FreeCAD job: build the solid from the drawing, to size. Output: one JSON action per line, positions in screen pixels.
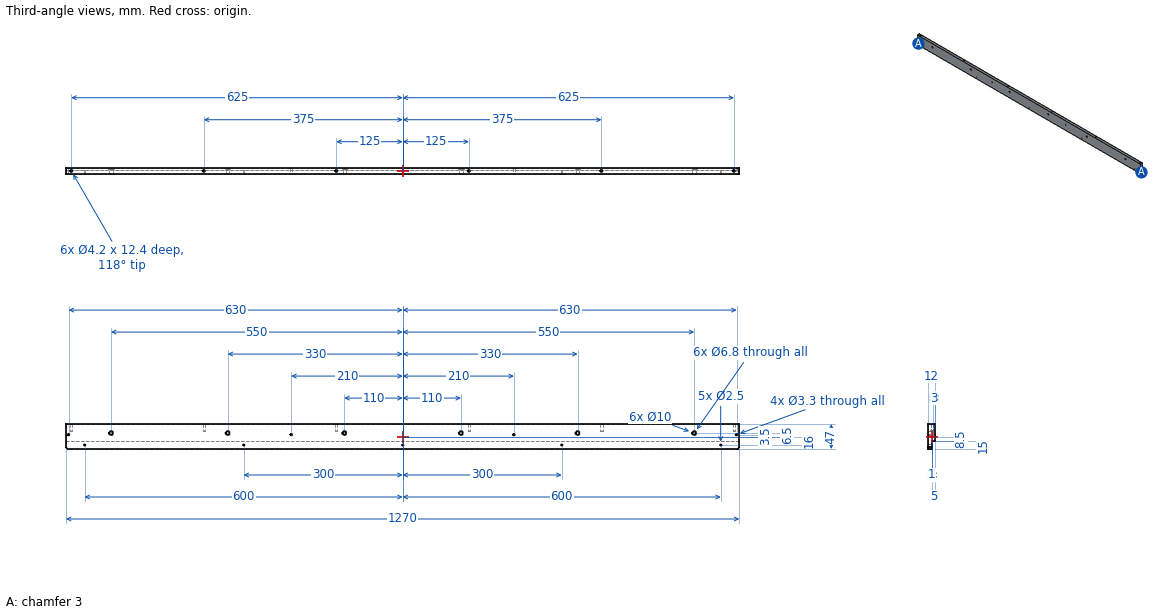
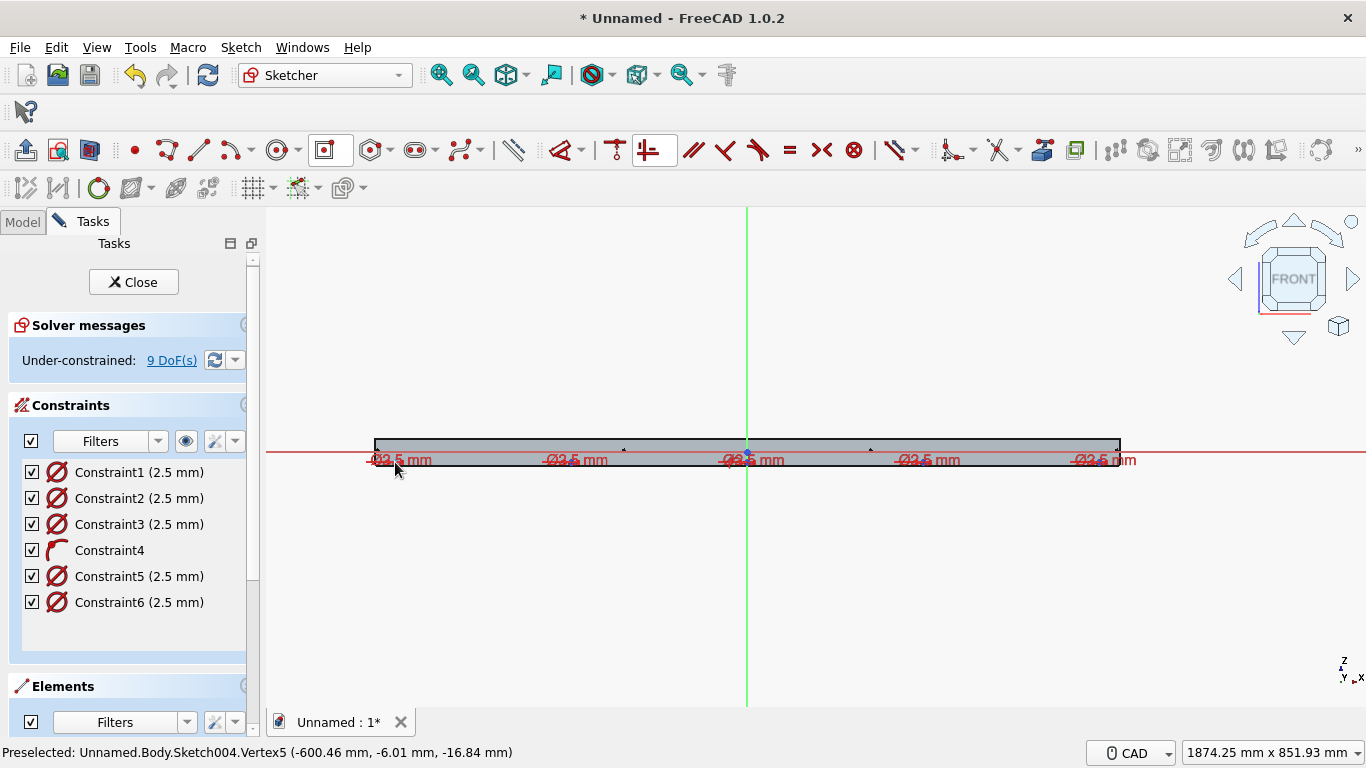
{"action": "left_click", "coordinate": [1100, 462]}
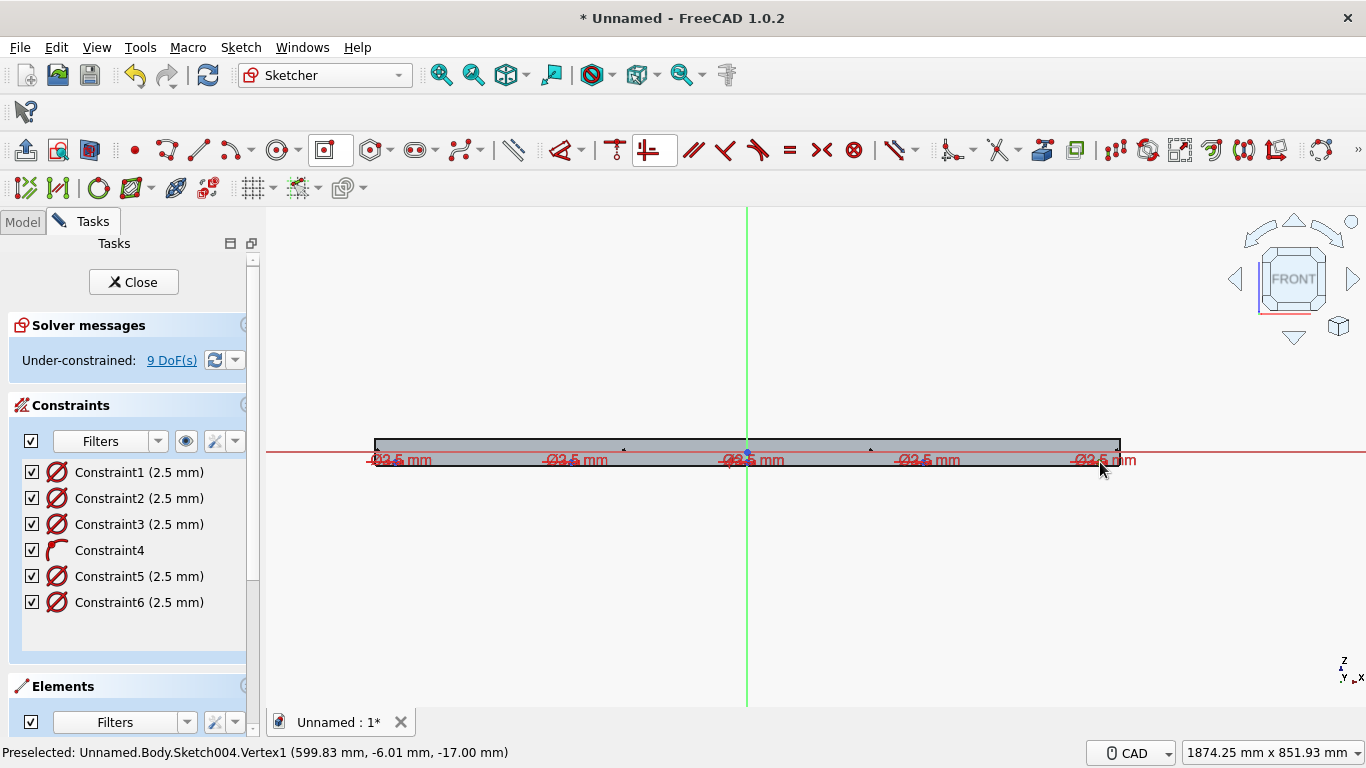
{"action": "left_click", "coordinate": [923, 462]}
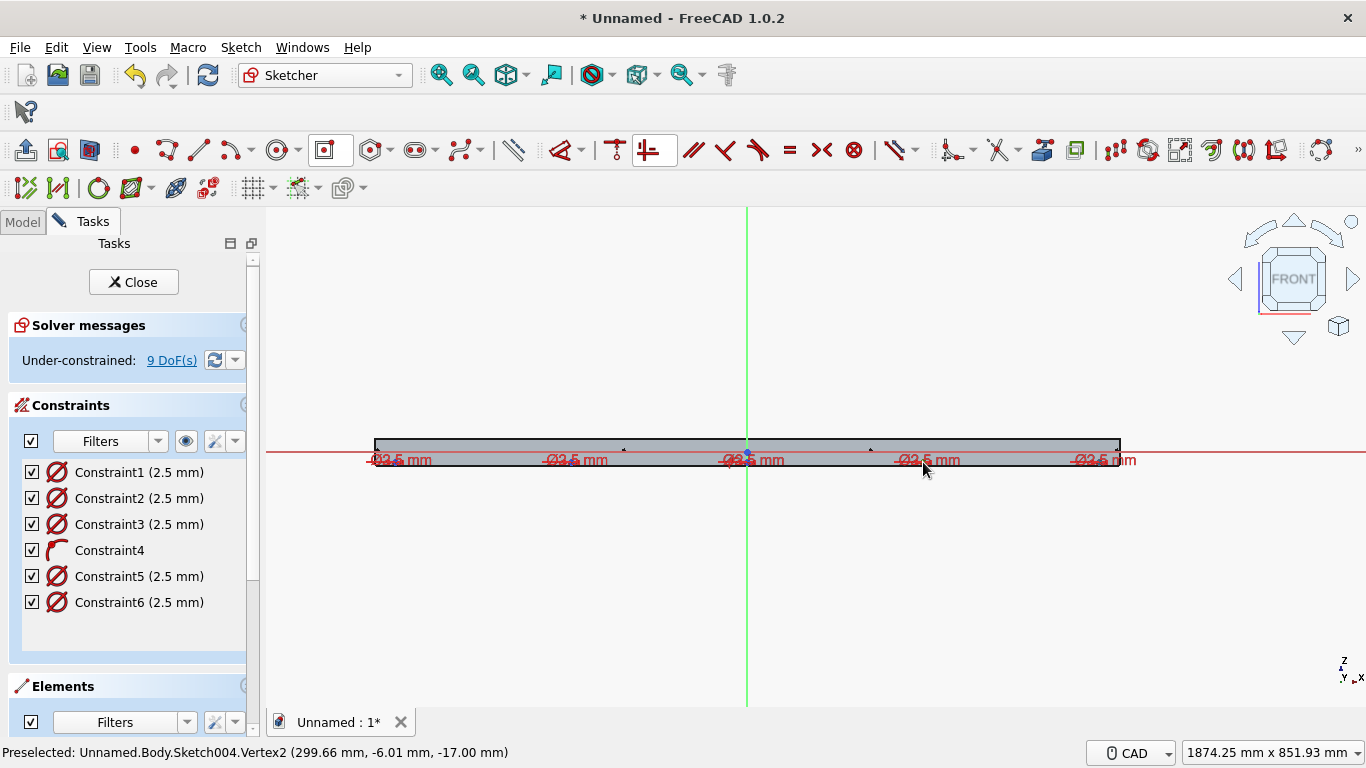
{"action": "key", "text": "h"}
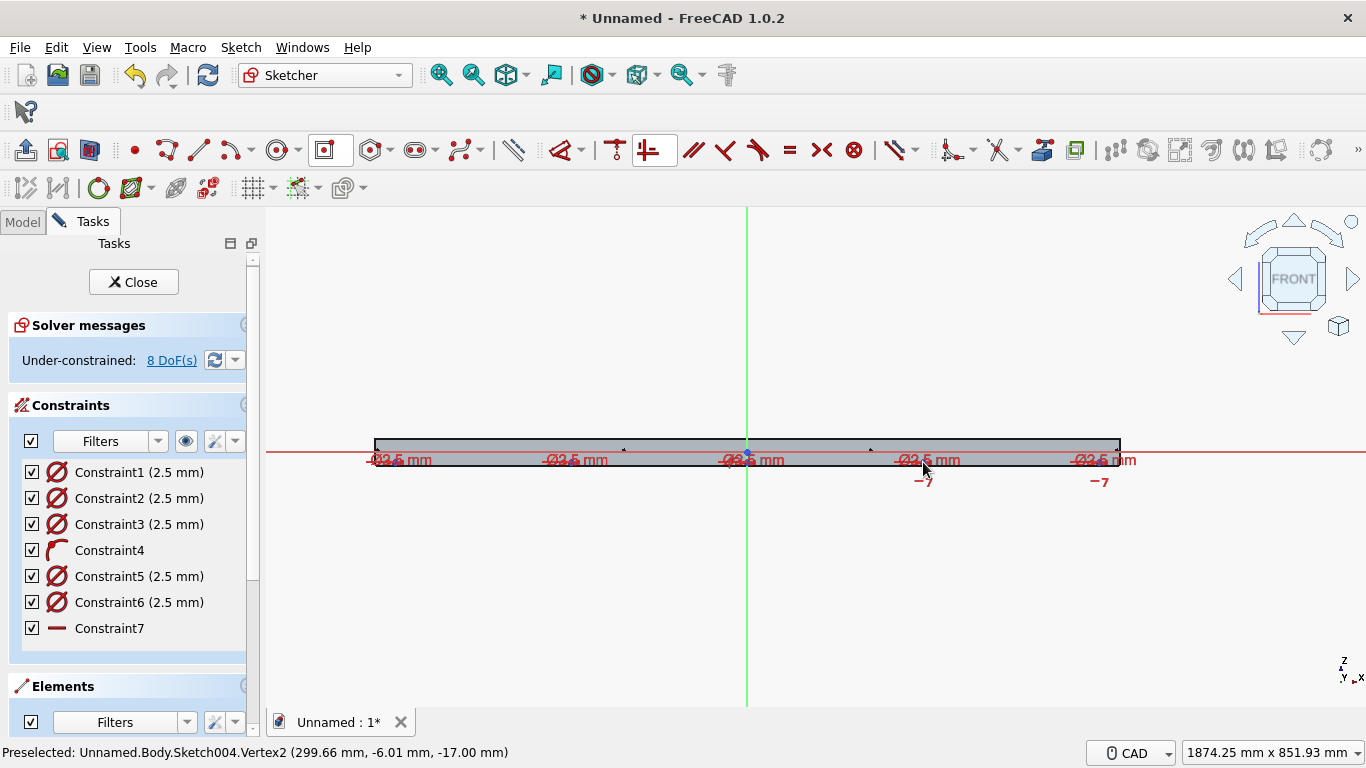
{"action": "left_click", "coordinate": [923, 462]}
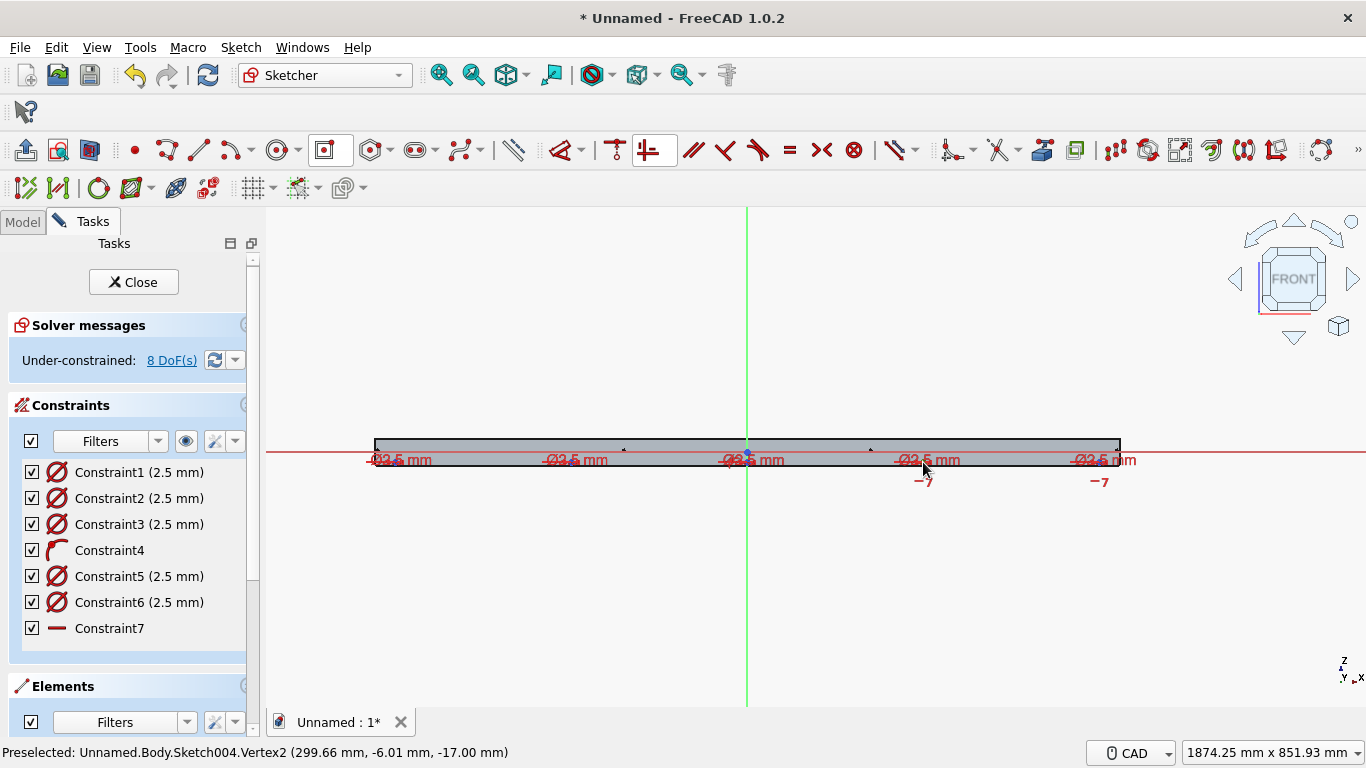
{"action": "scroll", "coordinate": [747, 462], "scroll_direction": "up", "scroll_amount": 2}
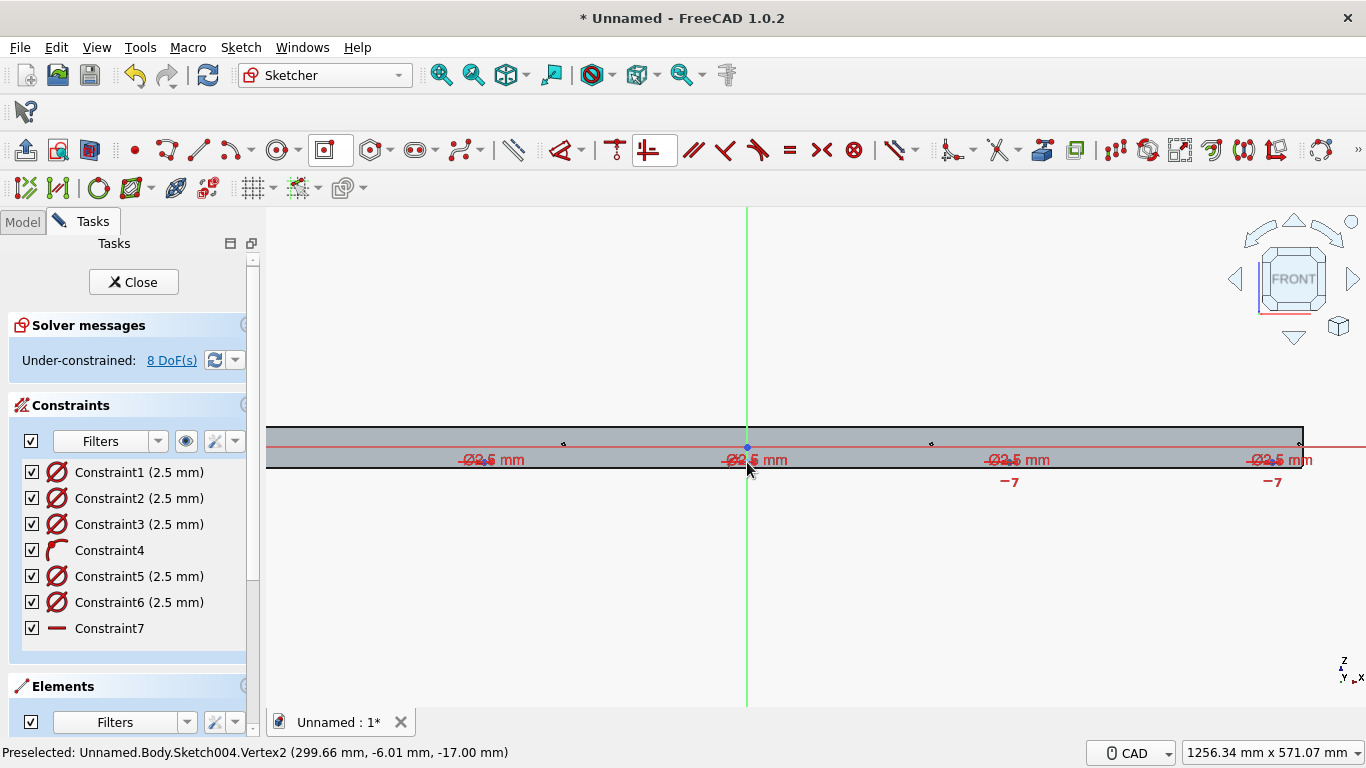
{"action": "left_click", "coordinate": [747, 462]}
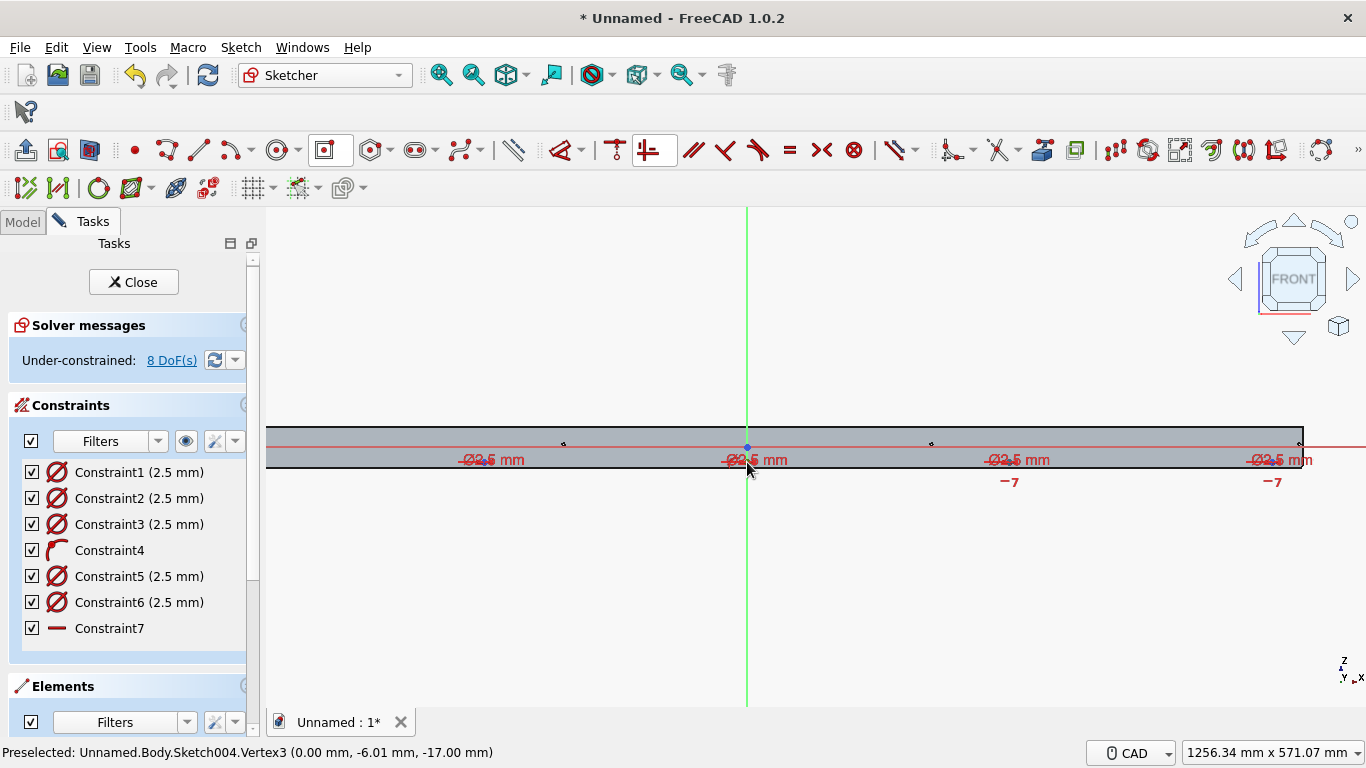
{"action": "left_click", "coordinate": [672, 150]}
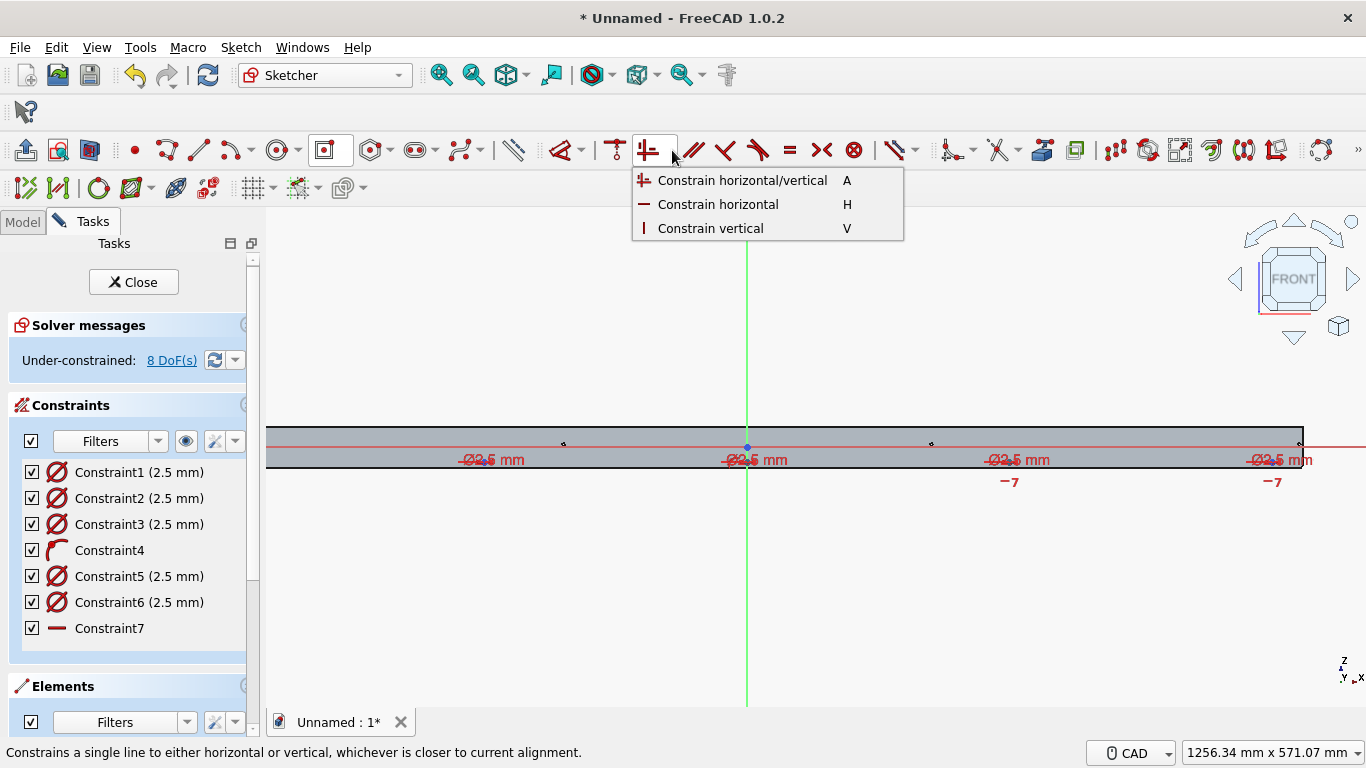
{"action": "left_click", "coordinate": [768, 204]}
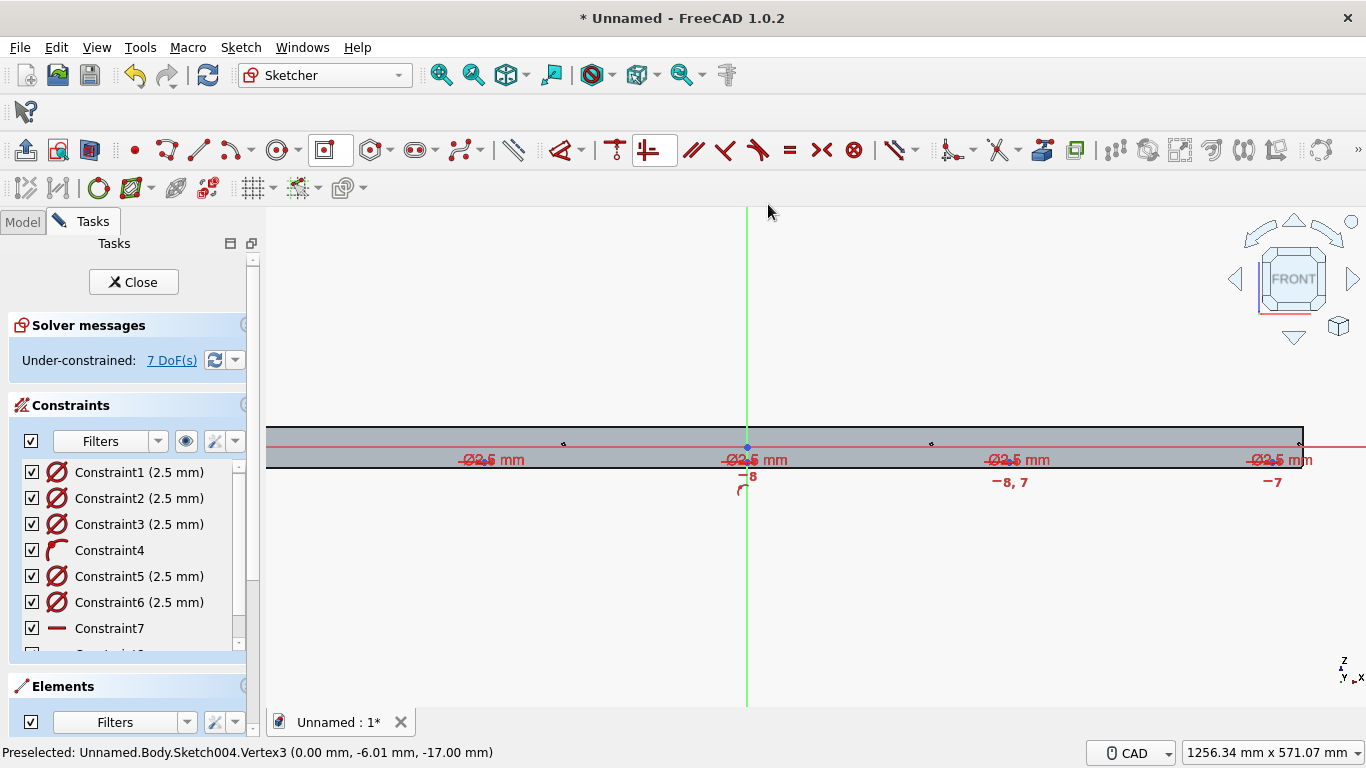
{"action": "left_click", "coordinate": [747, 462]}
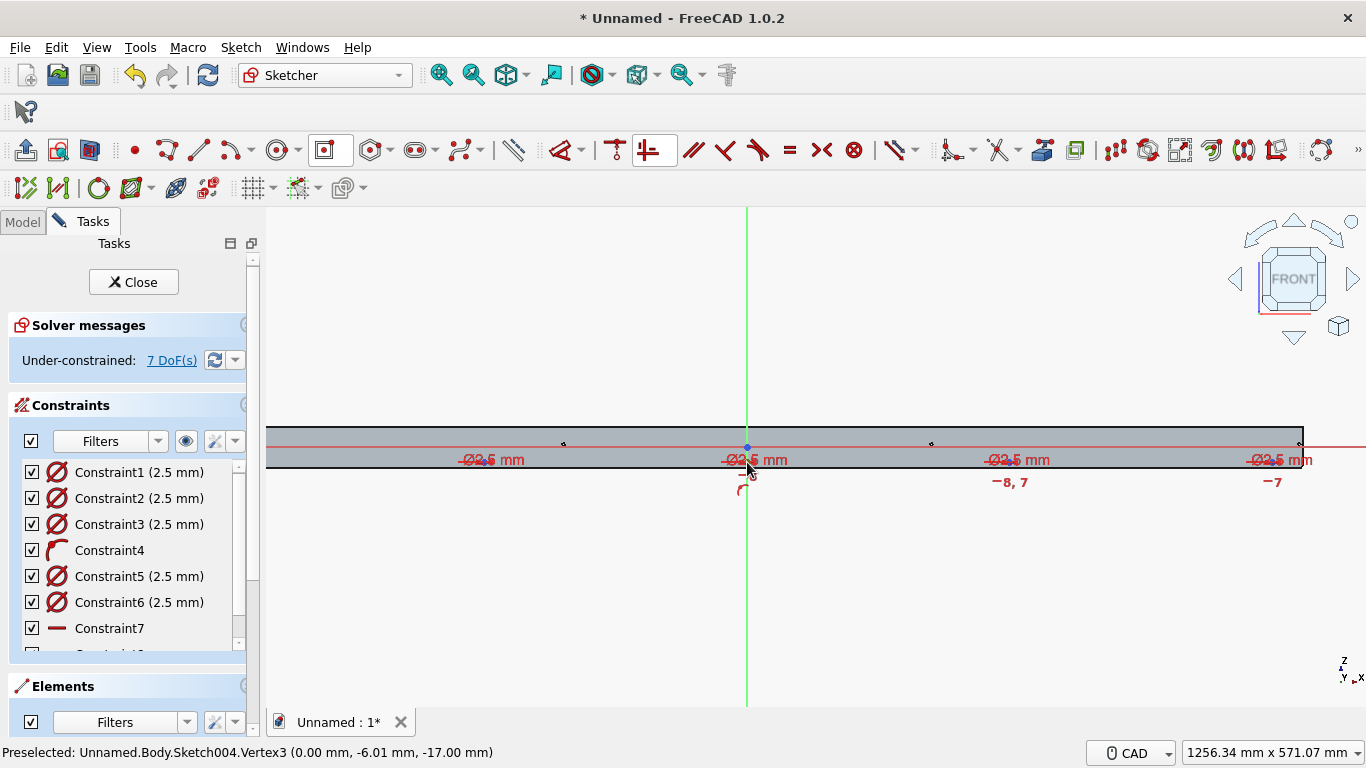
{"action": "left_click", "coordinate": [484, 462]}